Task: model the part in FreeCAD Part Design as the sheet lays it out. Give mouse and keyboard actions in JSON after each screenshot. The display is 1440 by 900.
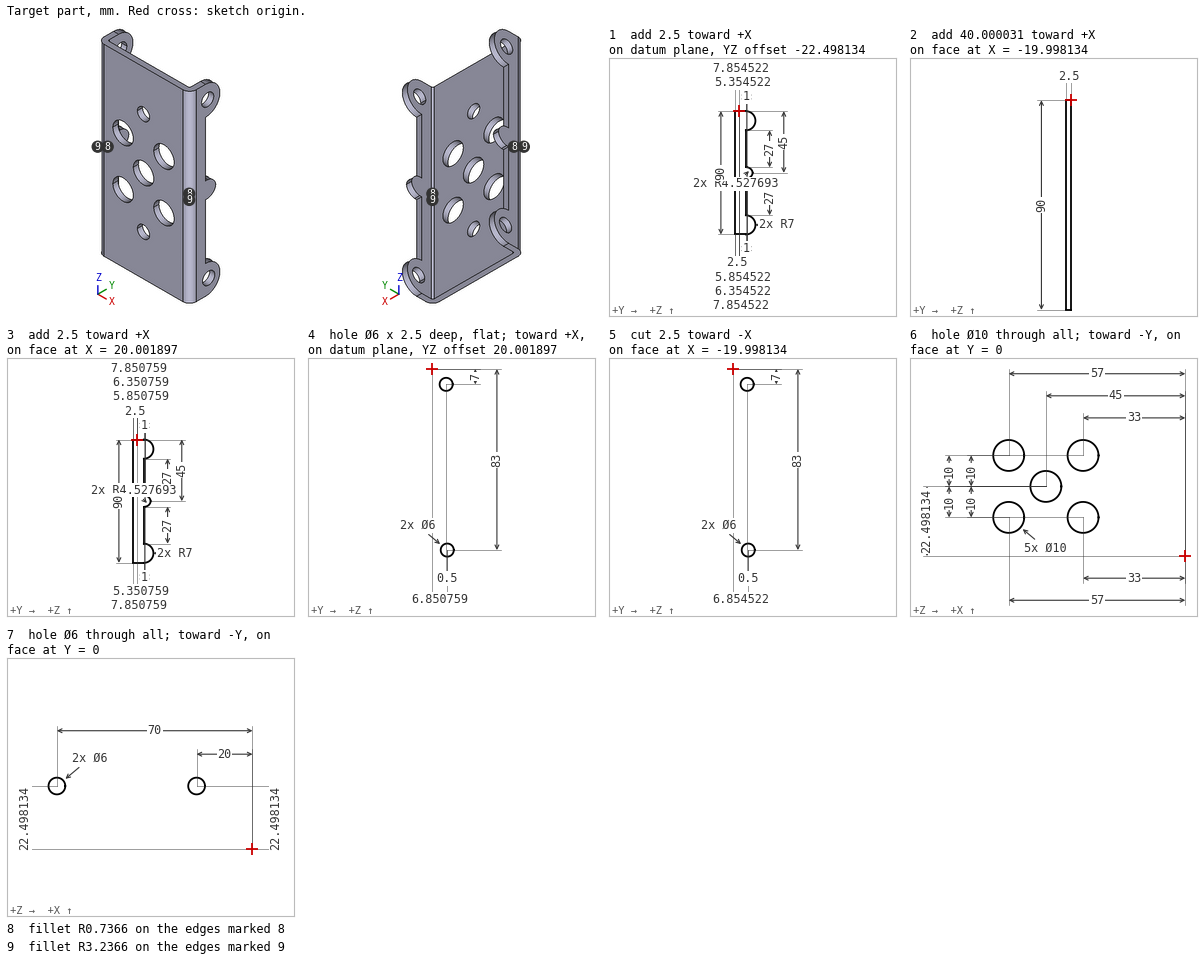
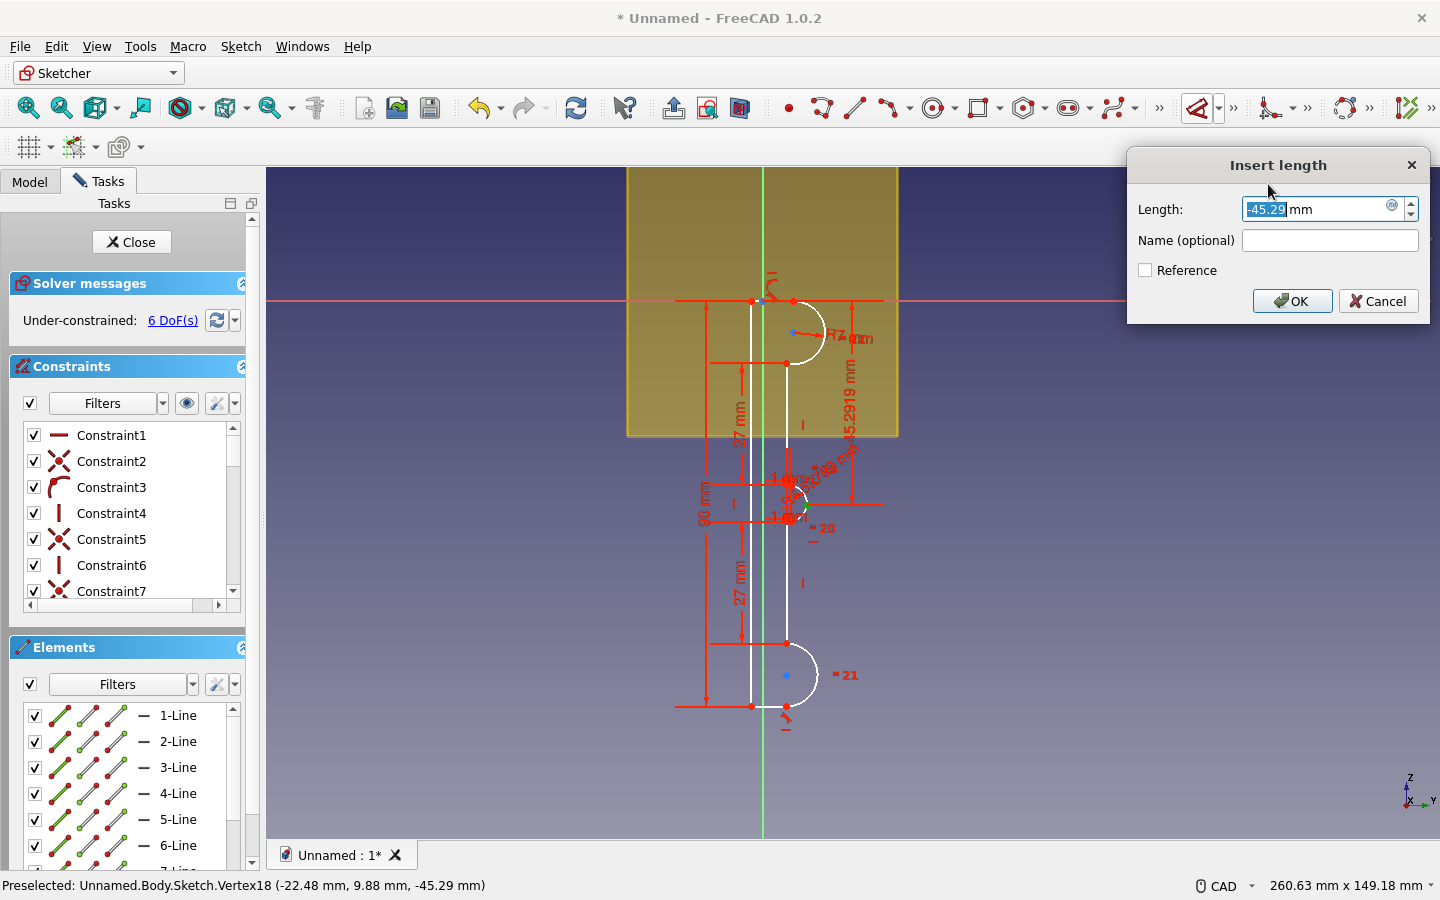
{"action": "type", "text": "-45"}
{"action": "key", "text": "Return"}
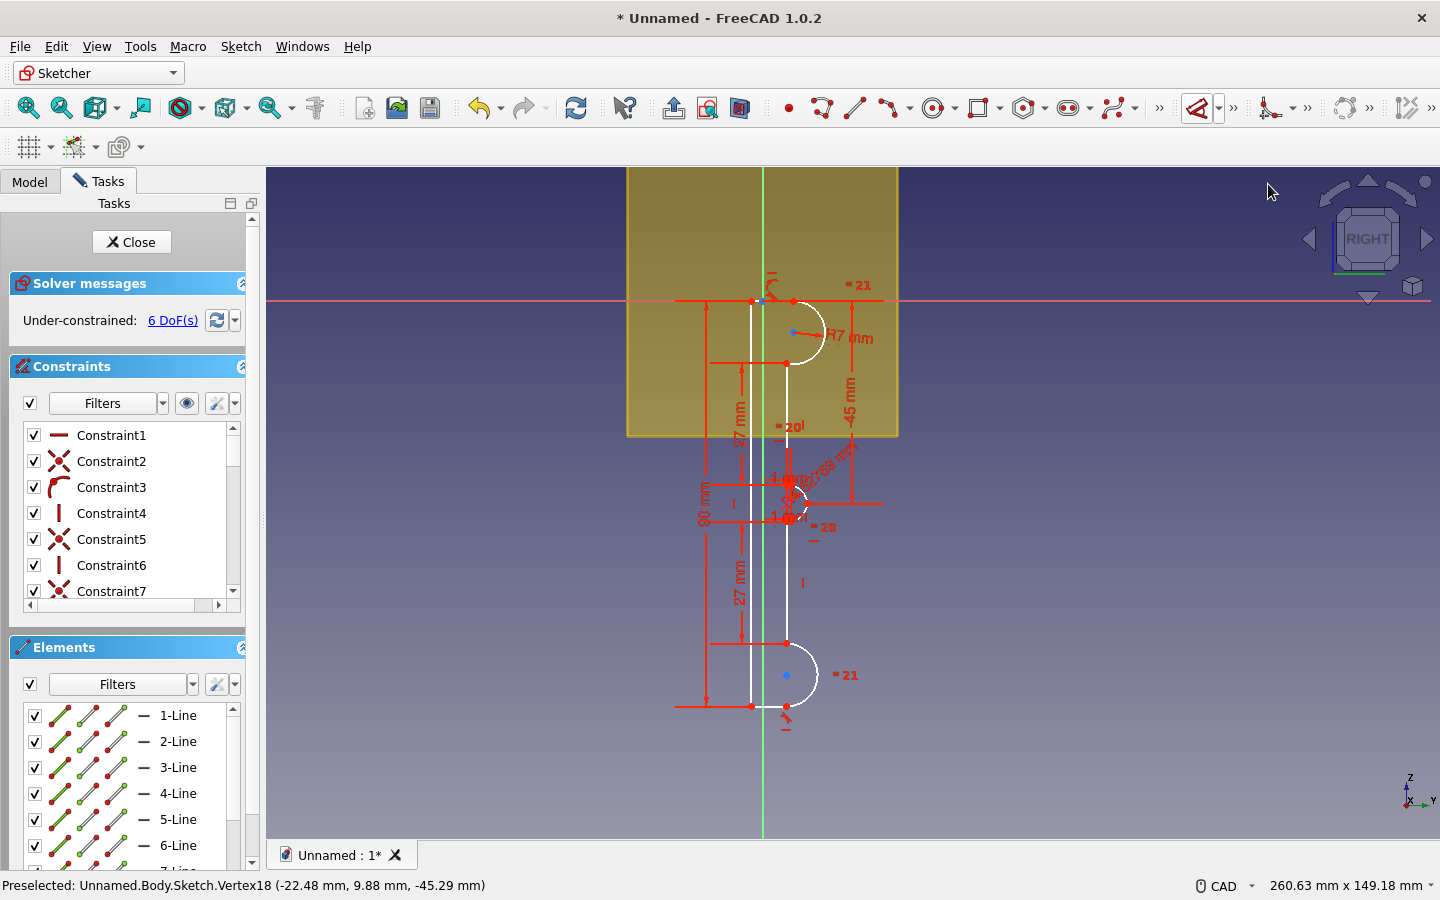
{"action": "scroll", "coordinate": [751, 707], "scroll_direction": "up", "scroll_amount": 7}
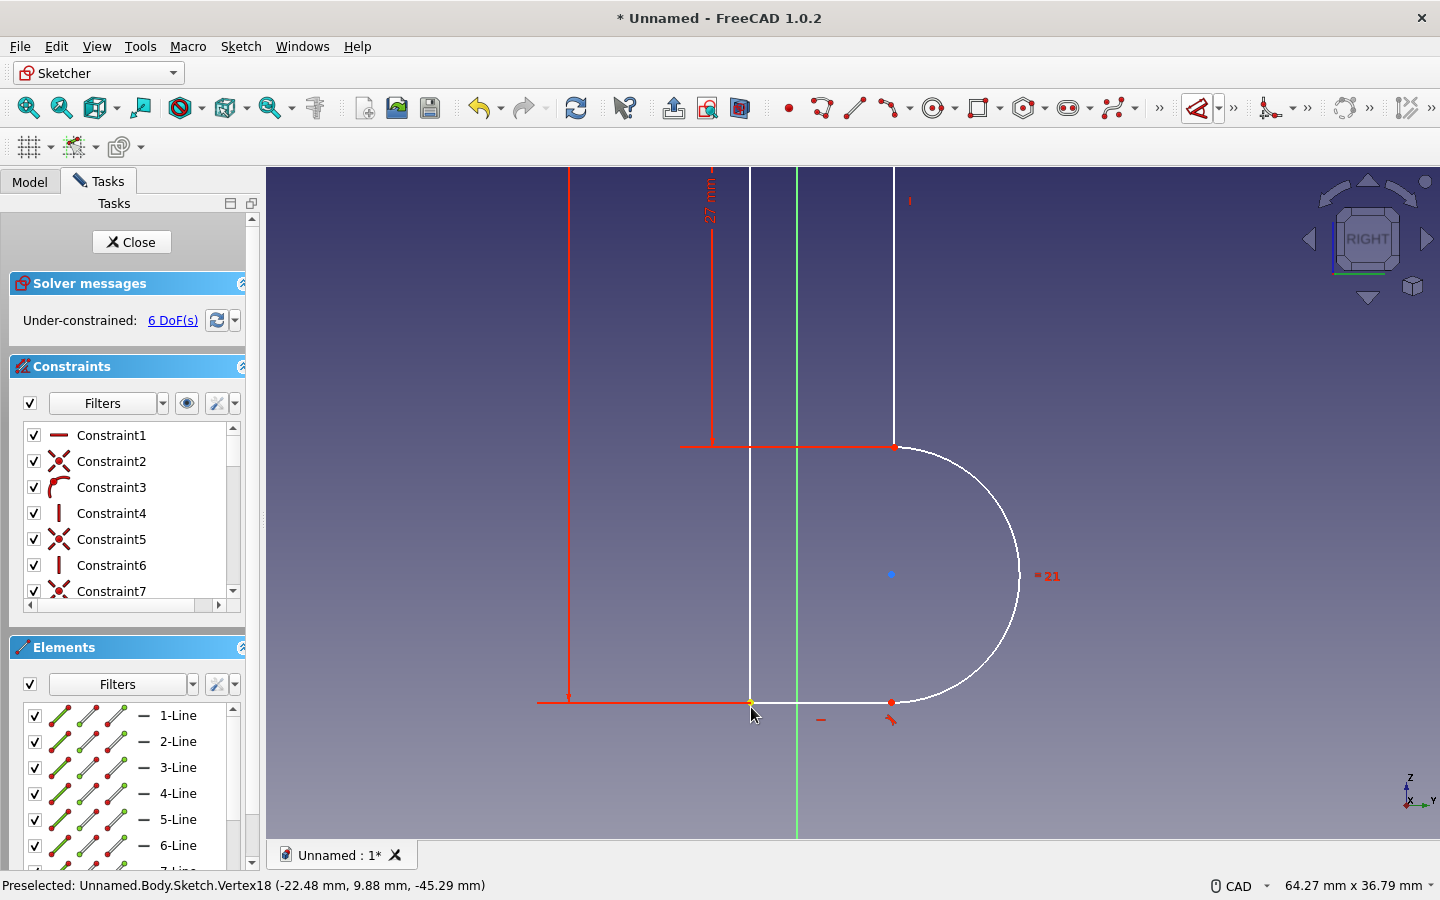
{"action": "left_click", "coordinate": [750, 703]}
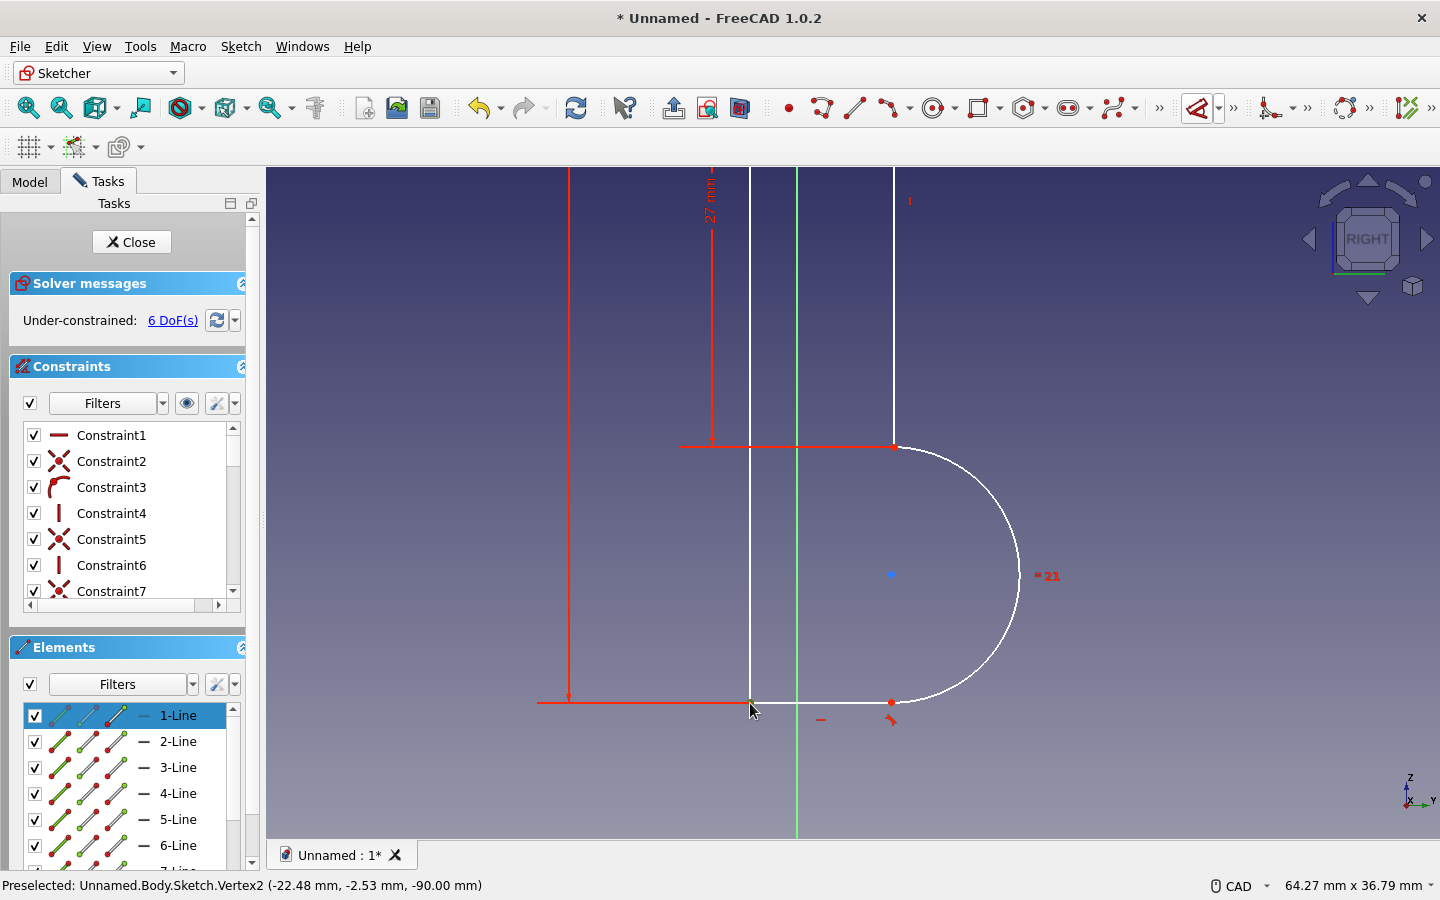
{"action": "key", "text": "l"}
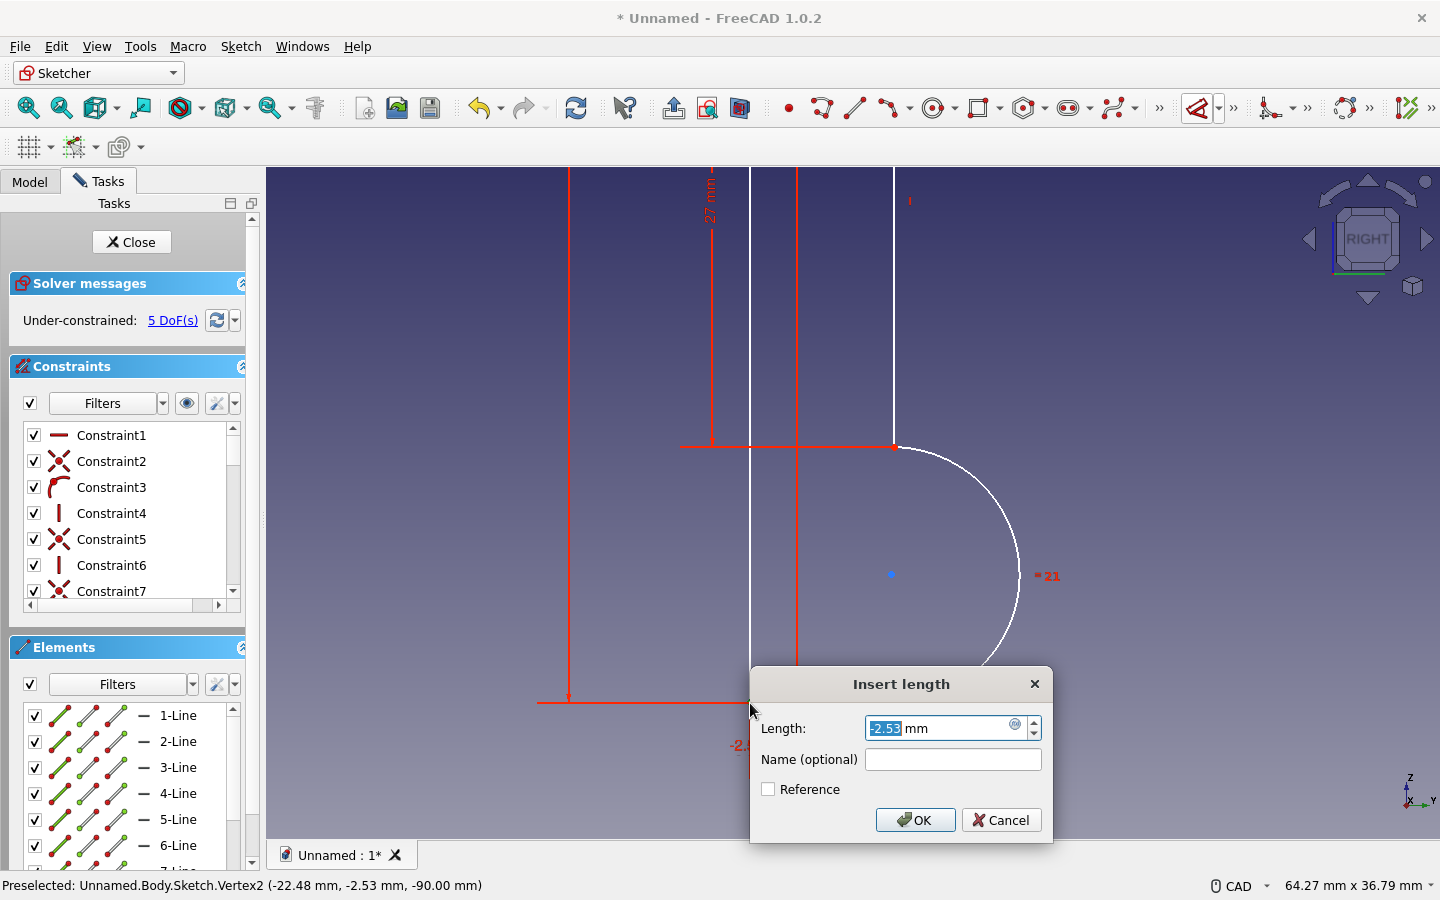
{"action": "type", "text": "-2.5"}
{"action": "key", "text": "Return"}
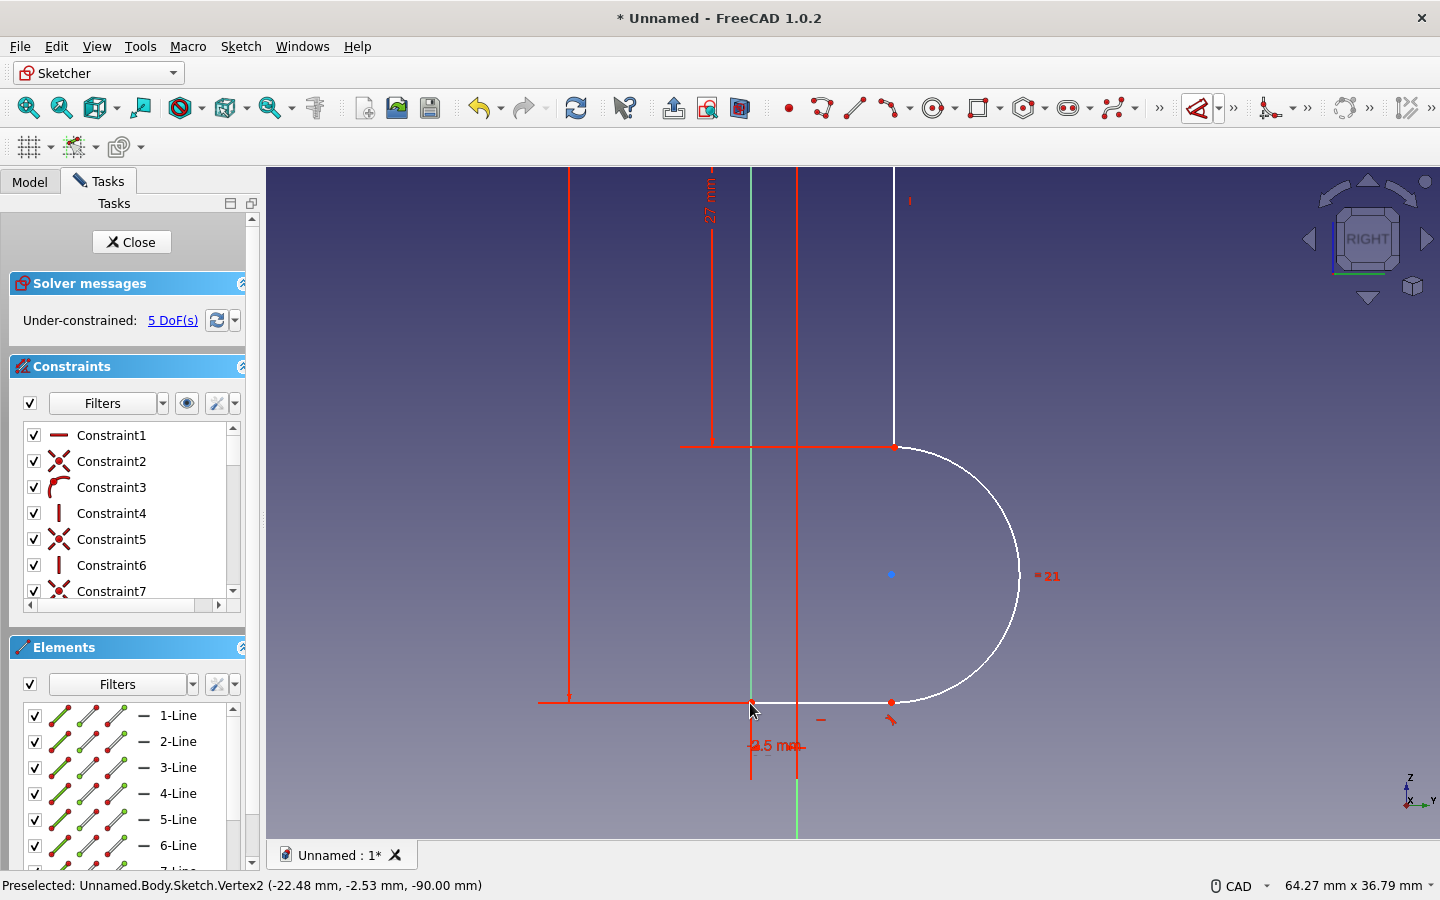
{"action": "scroll", "coordinate": [751, 707], "scroll_direction": "down", "scroll_amount": 7}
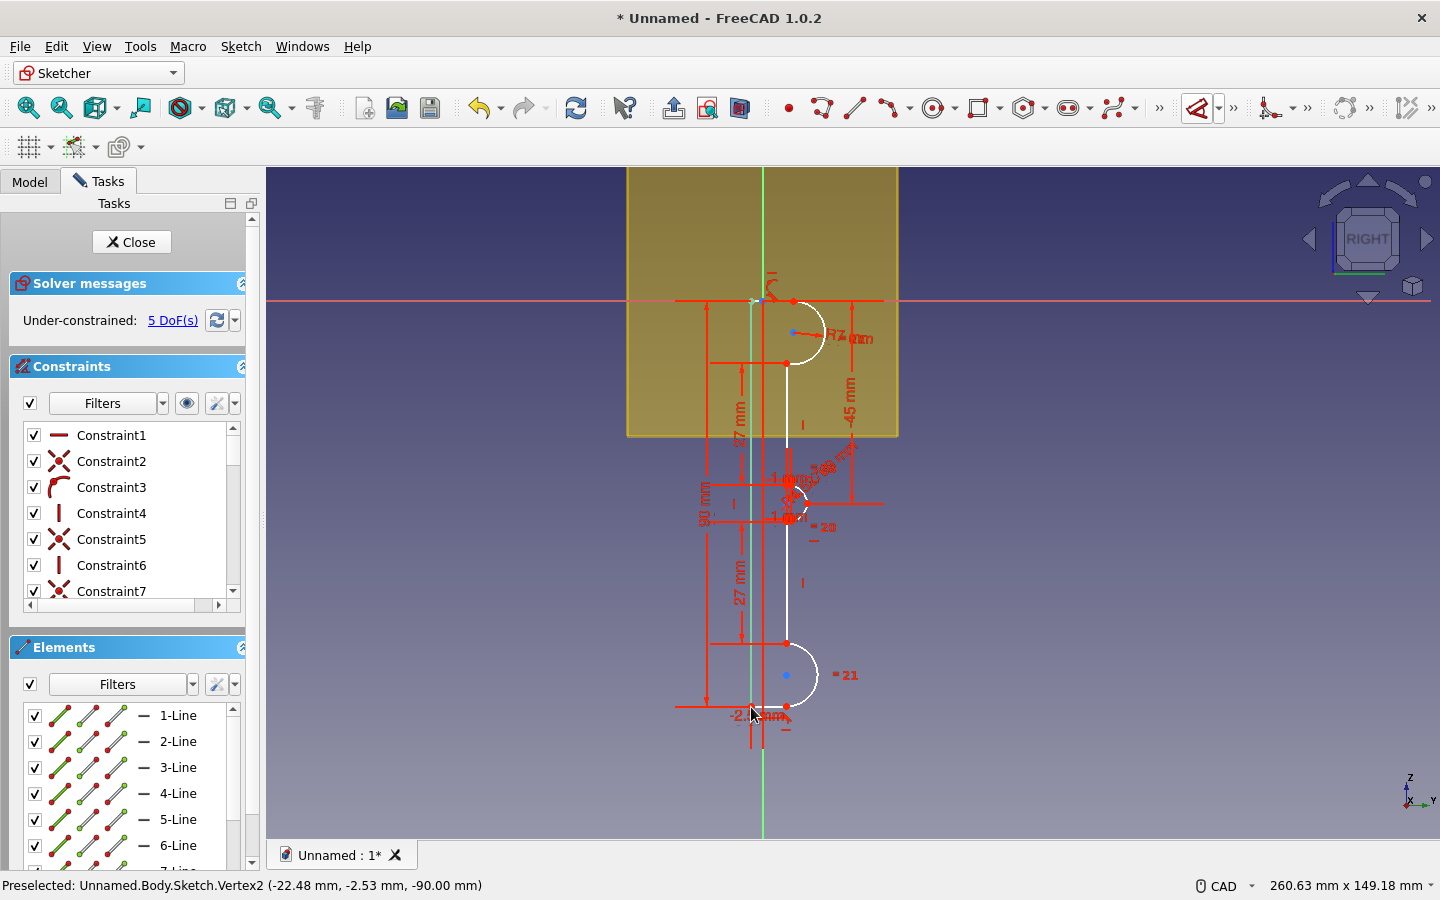
{"action": "scroll", "coordinate": [776, 707], "scroll_direction": "up", "scroll_amount": 2}